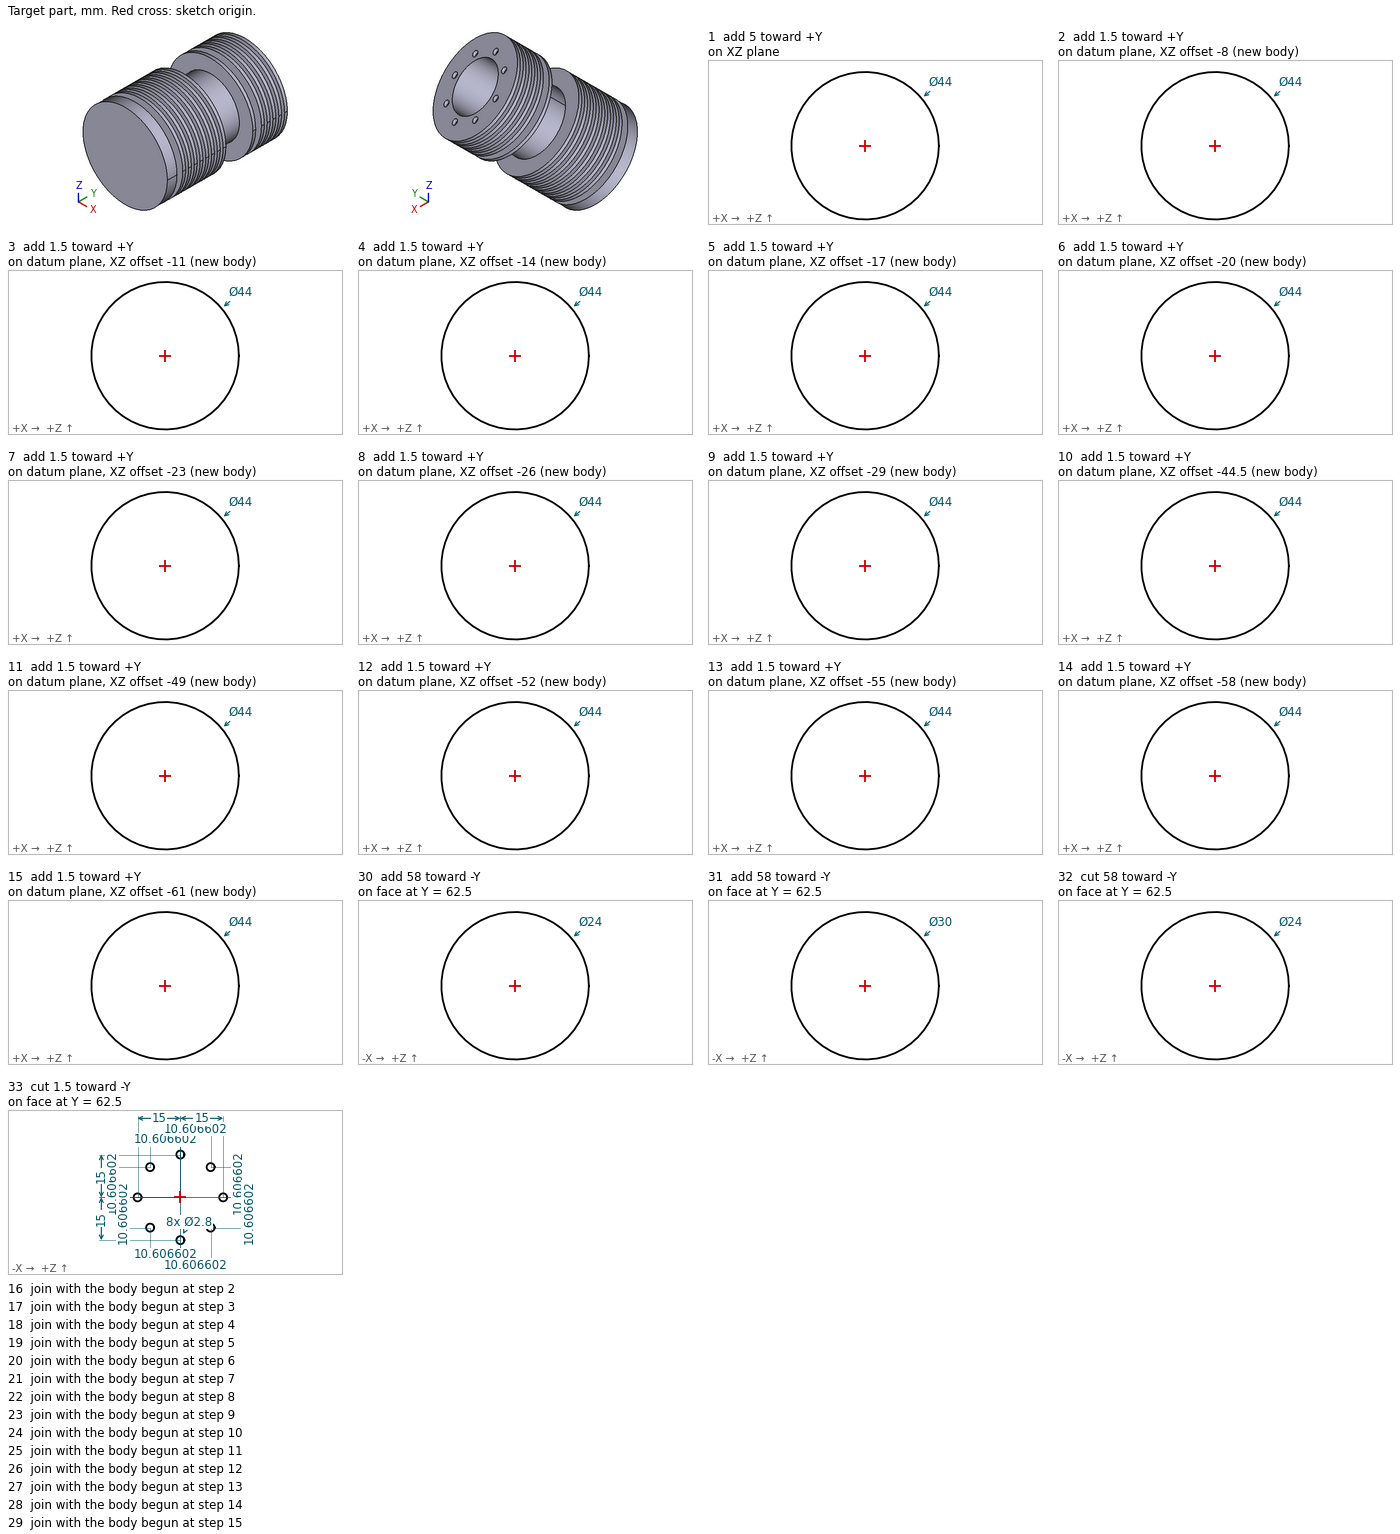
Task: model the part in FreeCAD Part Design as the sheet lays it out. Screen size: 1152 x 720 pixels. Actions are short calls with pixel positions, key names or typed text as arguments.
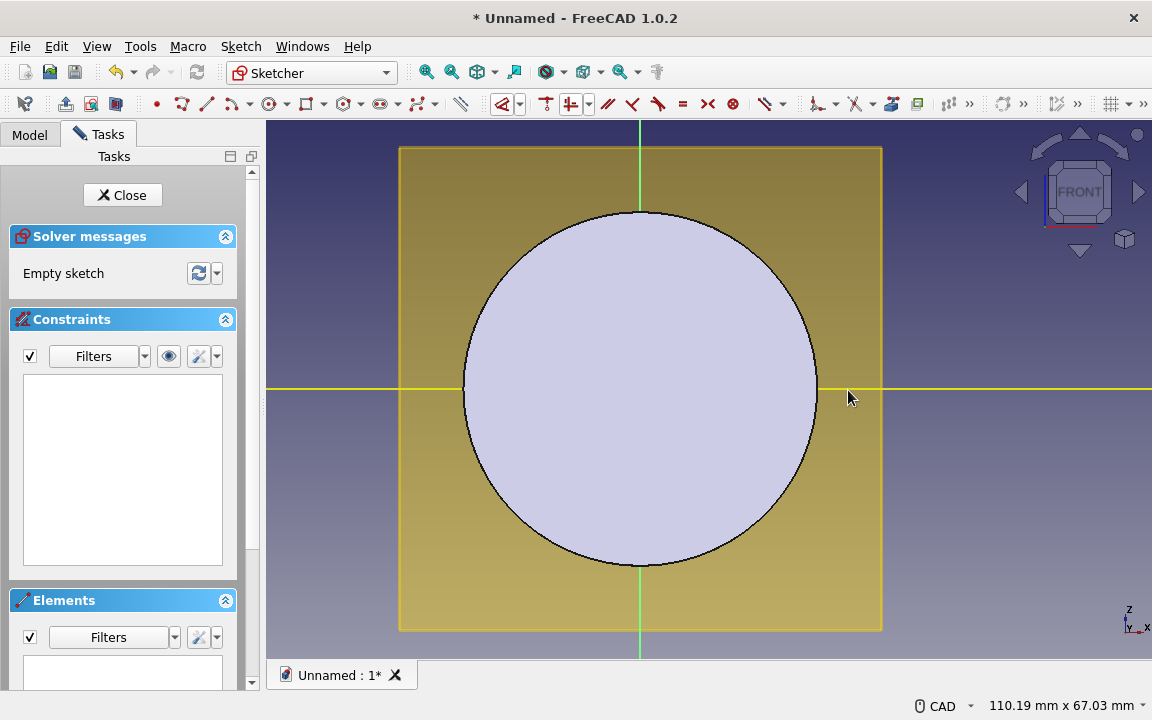
click(268, 104)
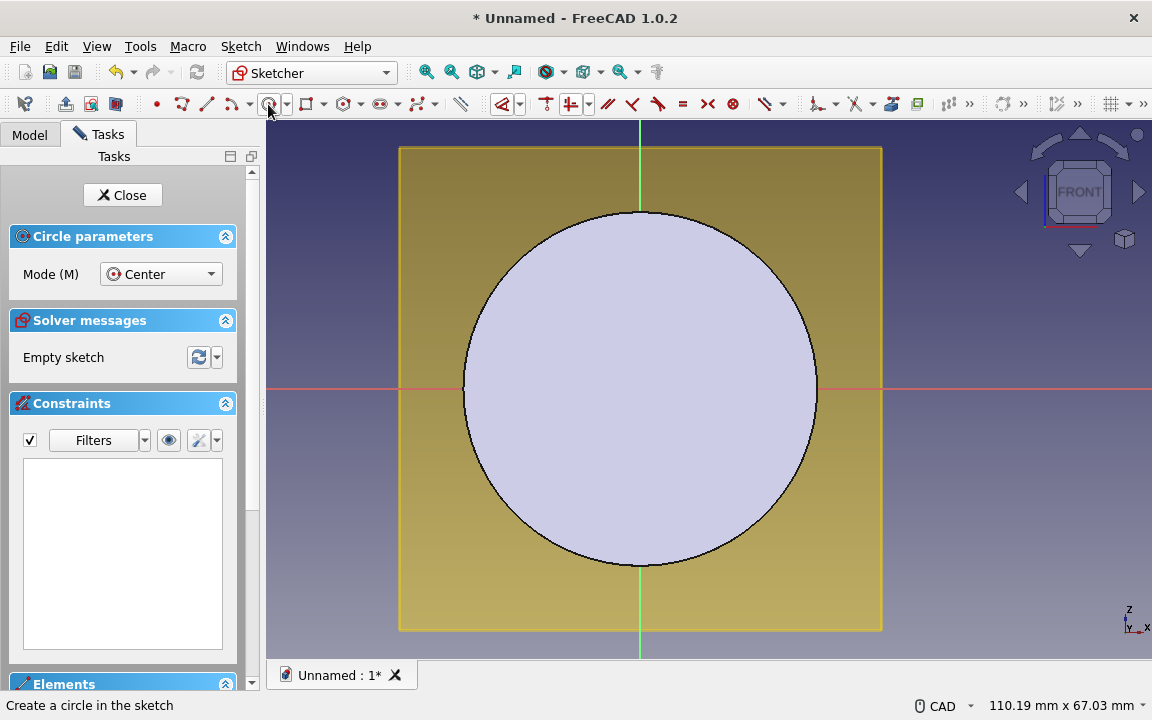
click(640, 389)
click(765, 264)
key(Escape)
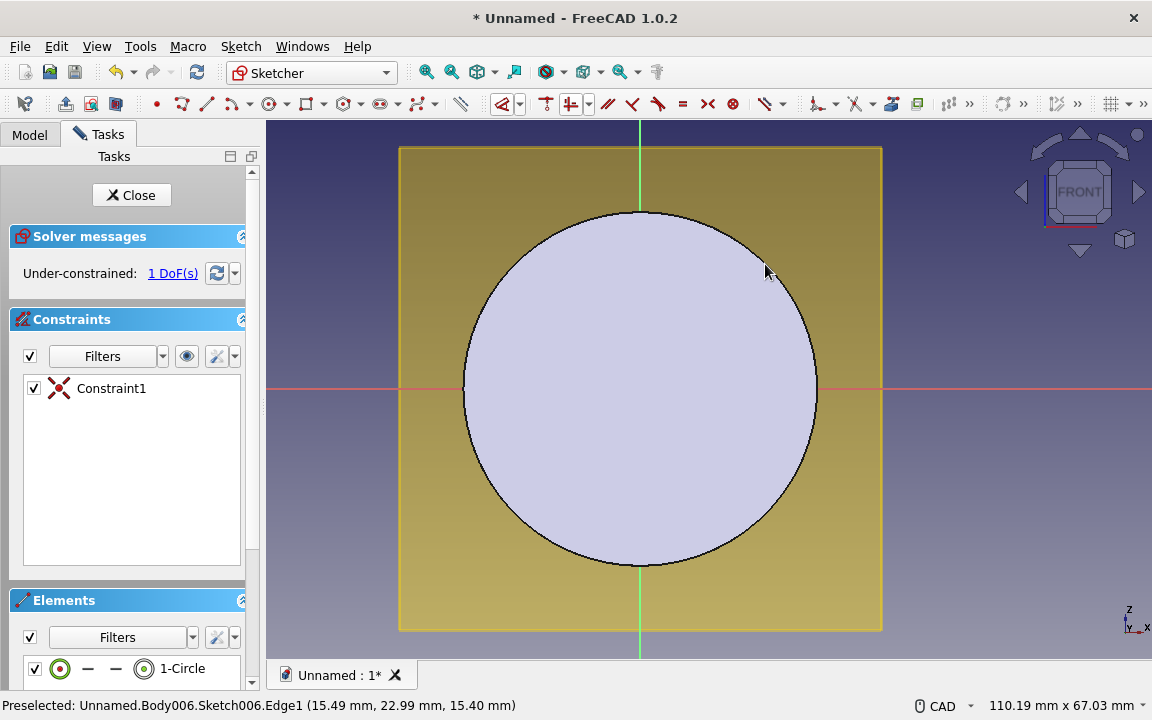
click(764, 264)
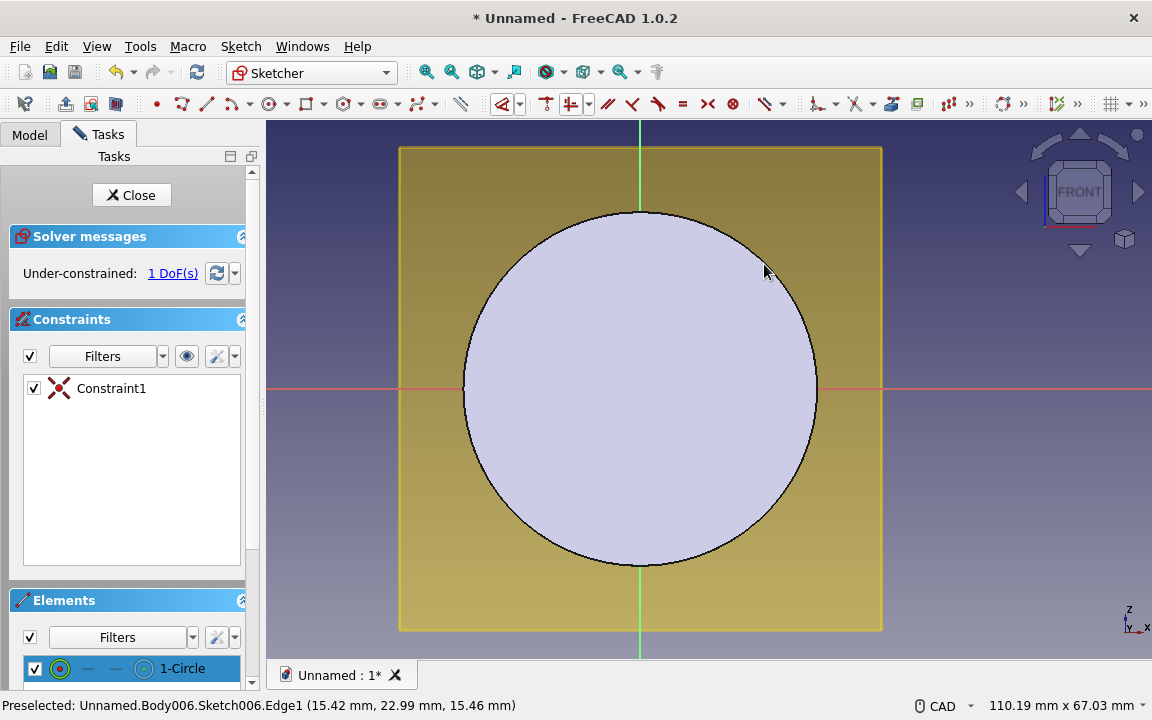
key(k)
key(o)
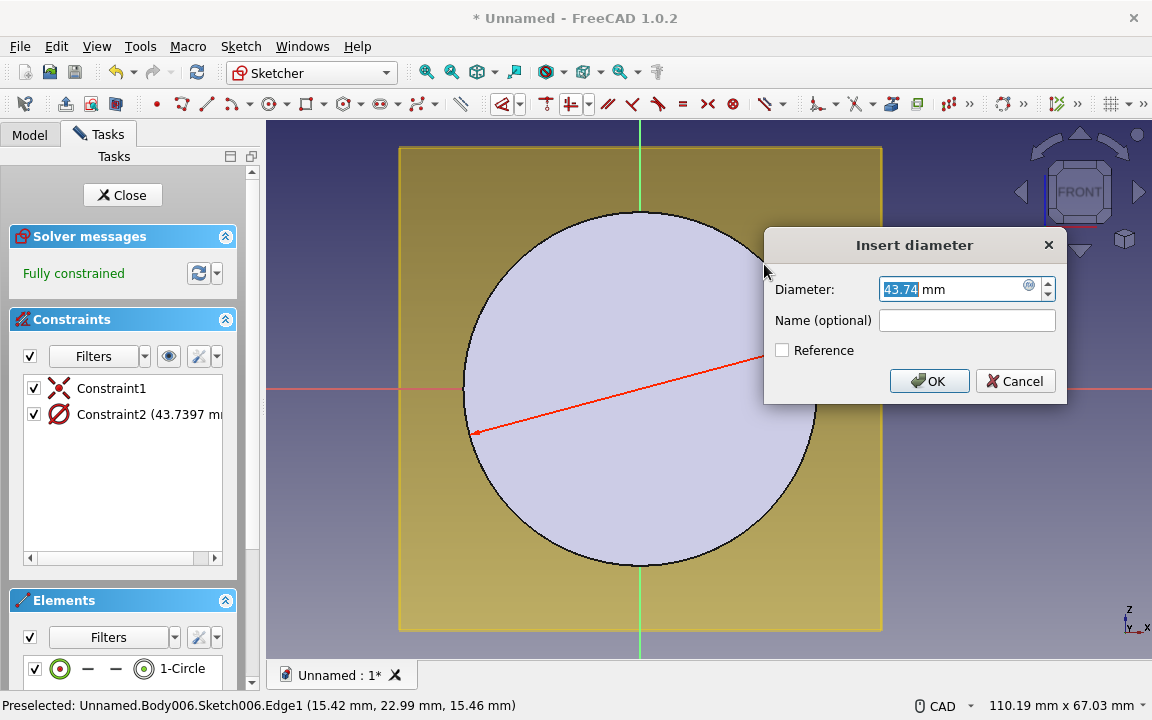
text(44)
key(Return)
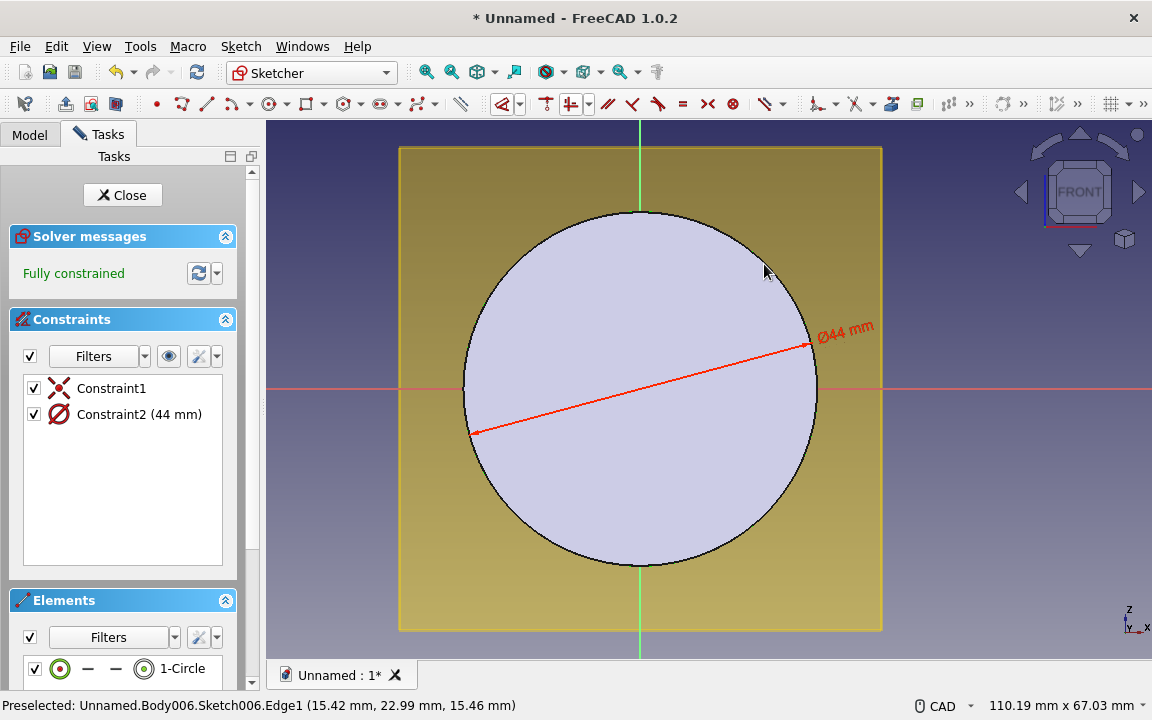
click(123, 195)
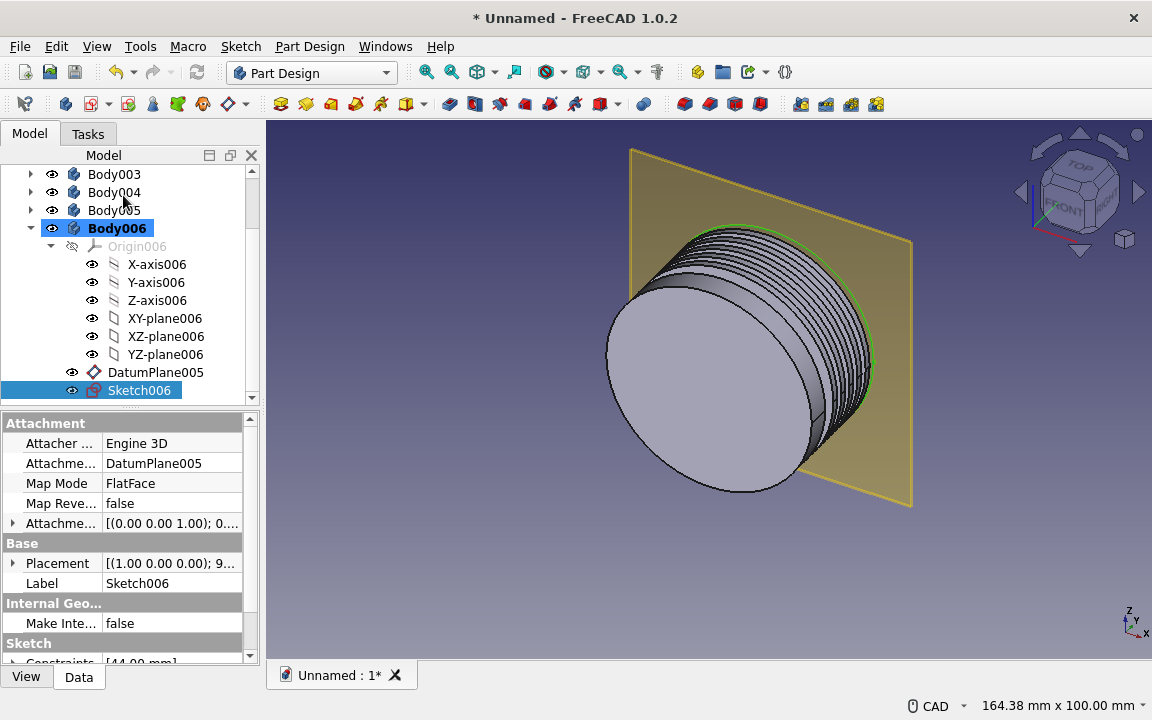
click(281, 104)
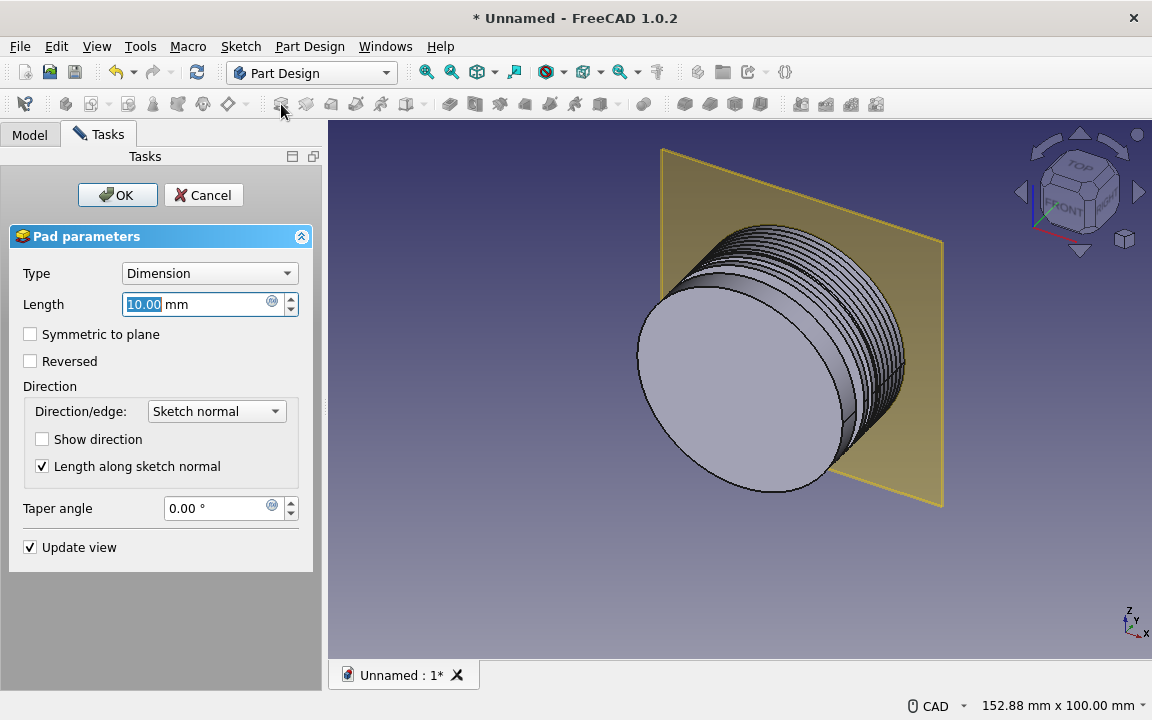
text(1.5)
key(Tab)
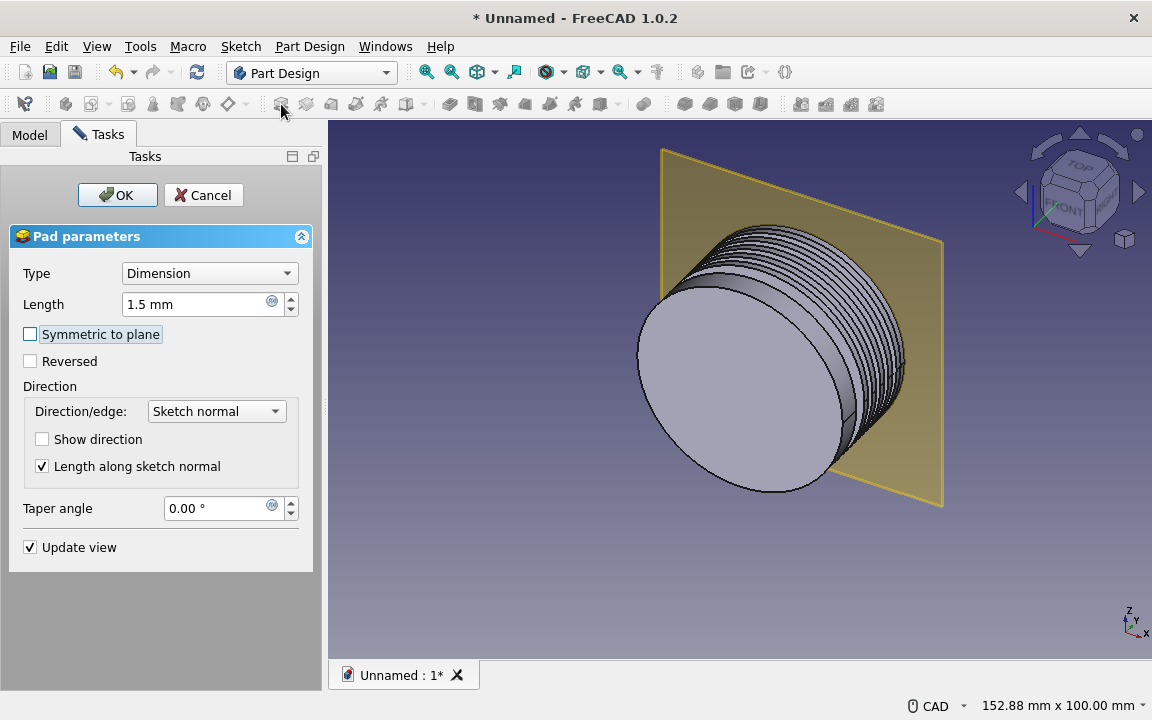
click(31, 361)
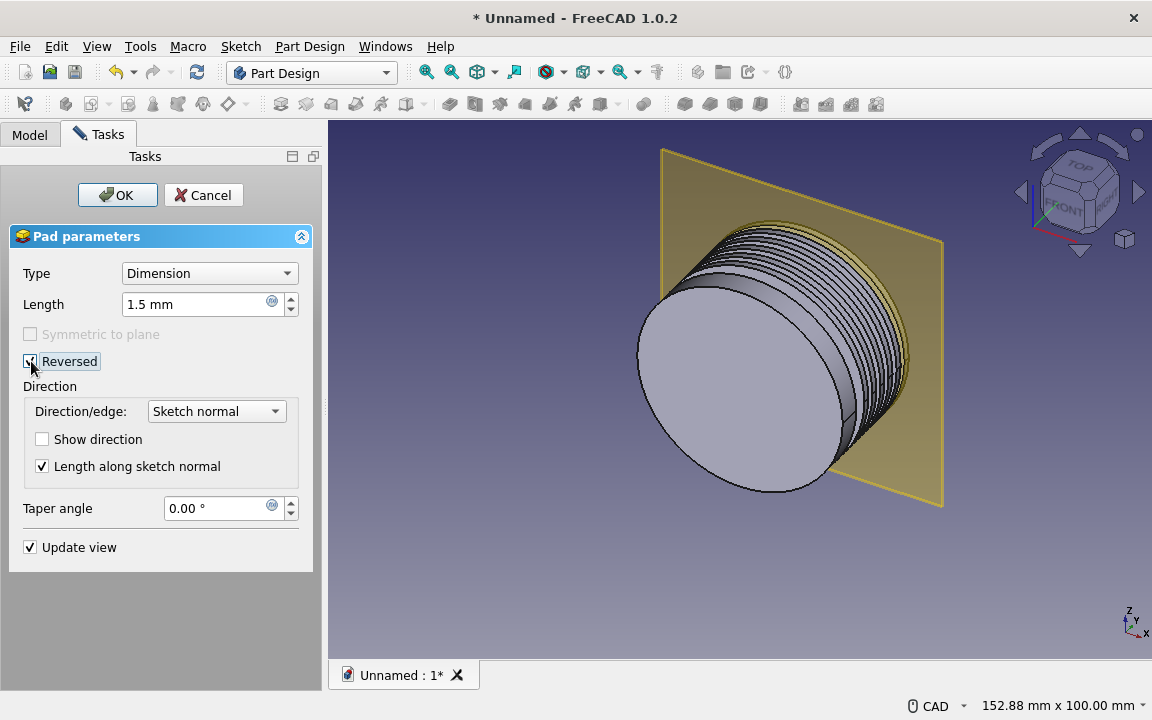
click(118, 195)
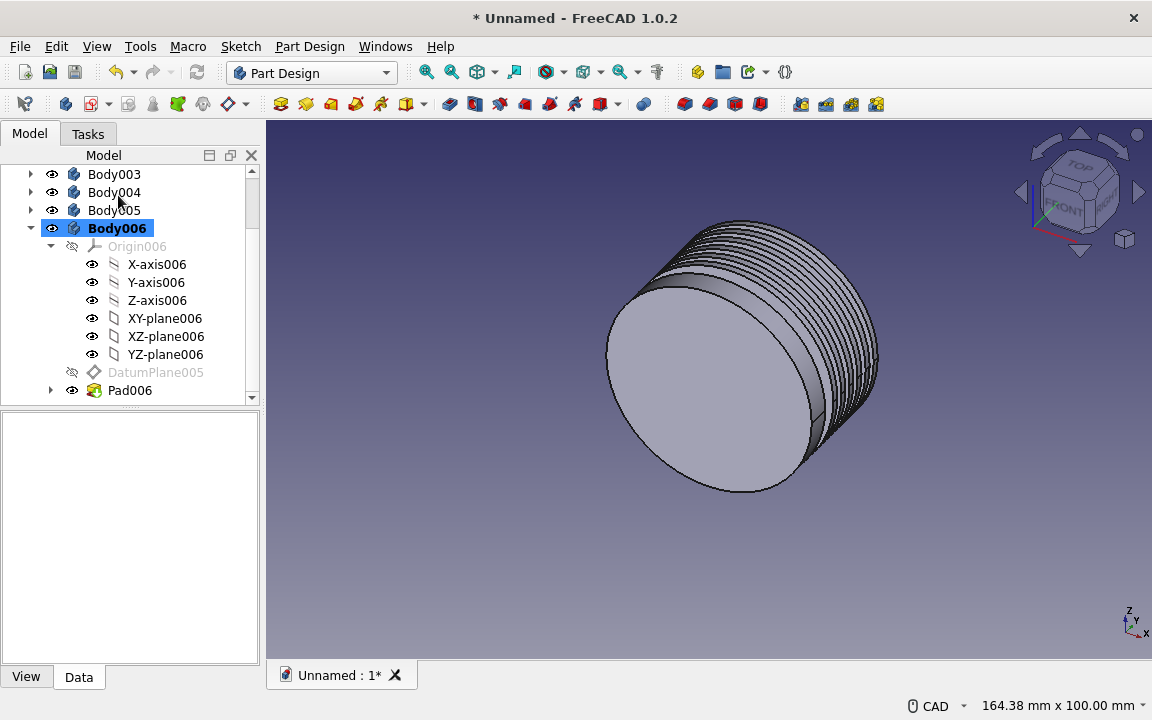
click(66, 104)